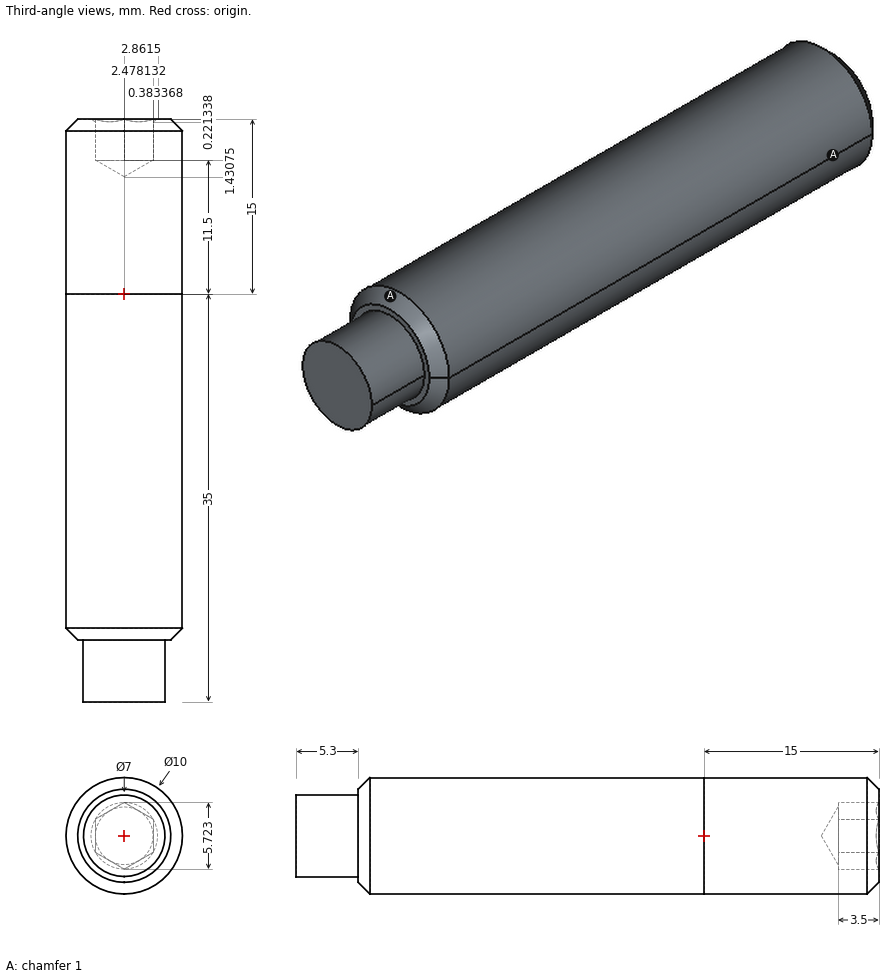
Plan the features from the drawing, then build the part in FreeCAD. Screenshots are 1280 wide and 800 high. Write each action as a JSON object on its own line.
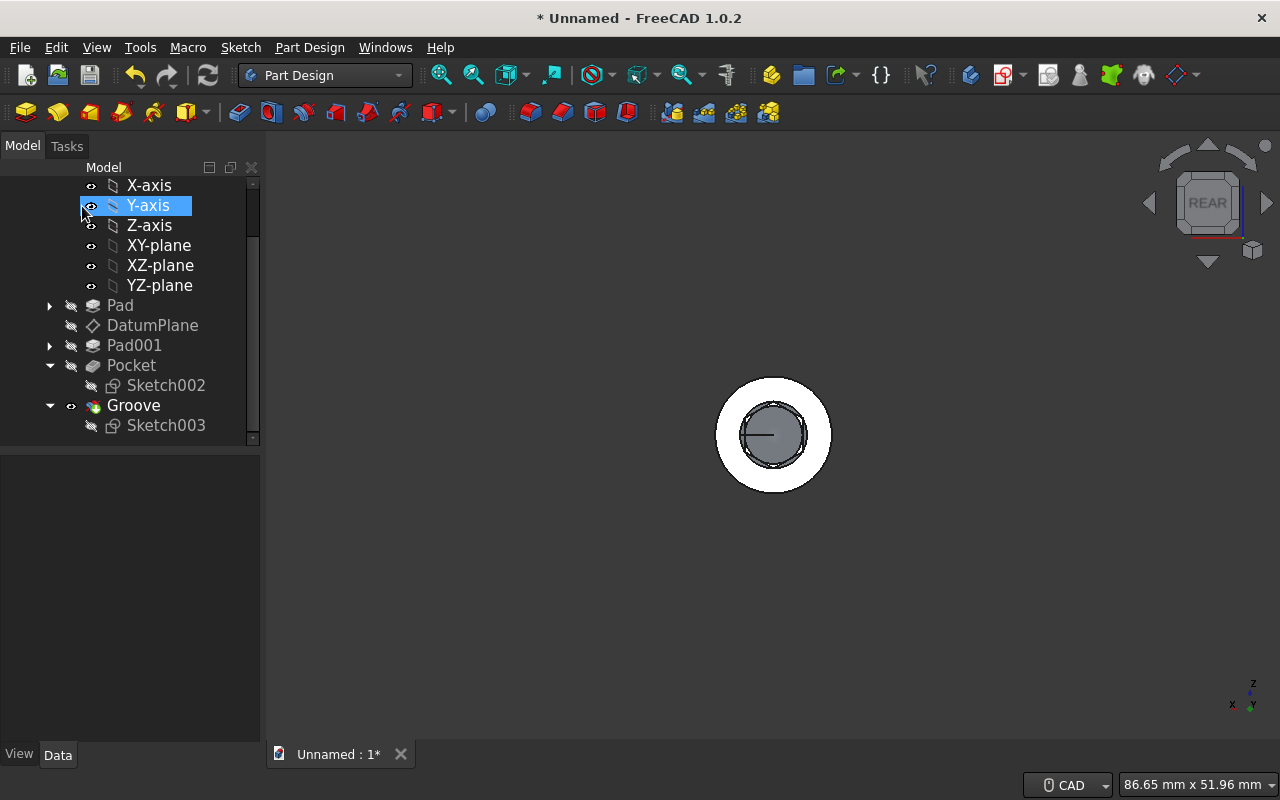
{"action": "left_click", "coordinate": [442, 76]}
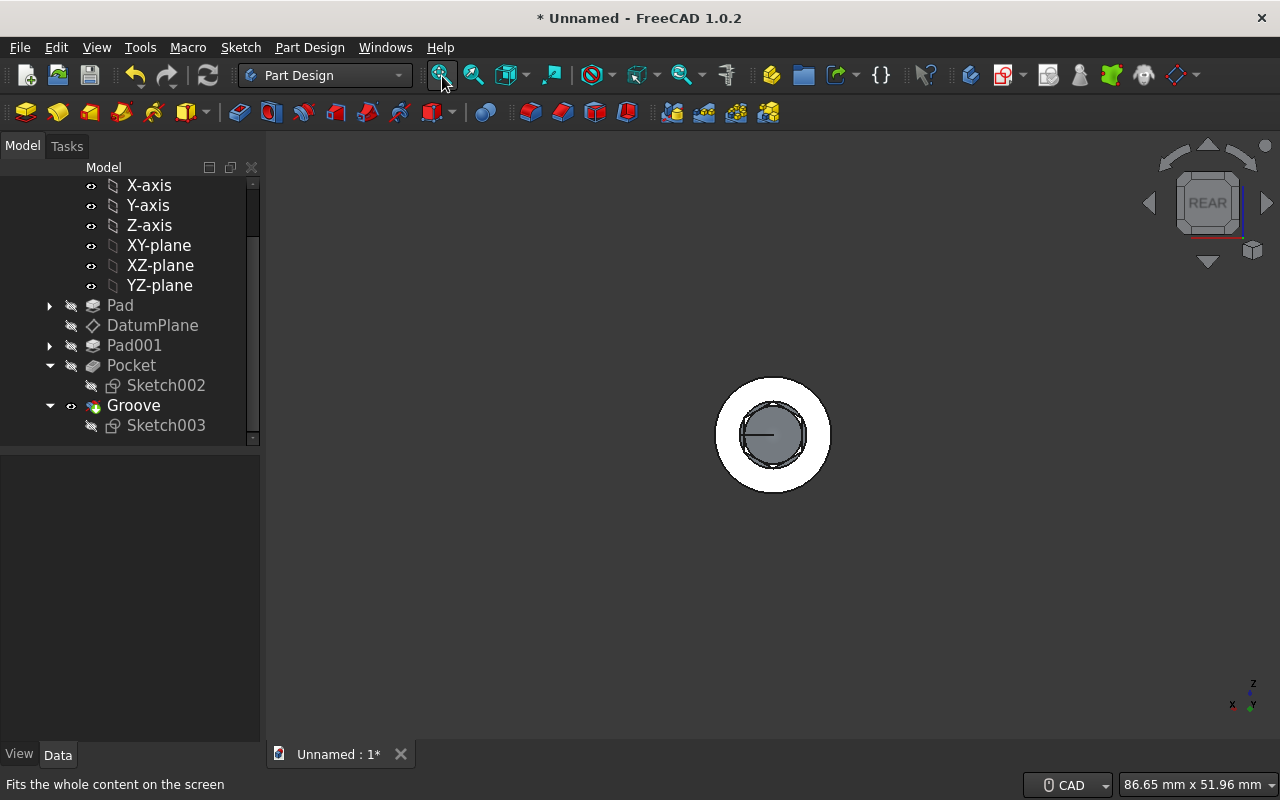
{"action": "key", "text": "0"}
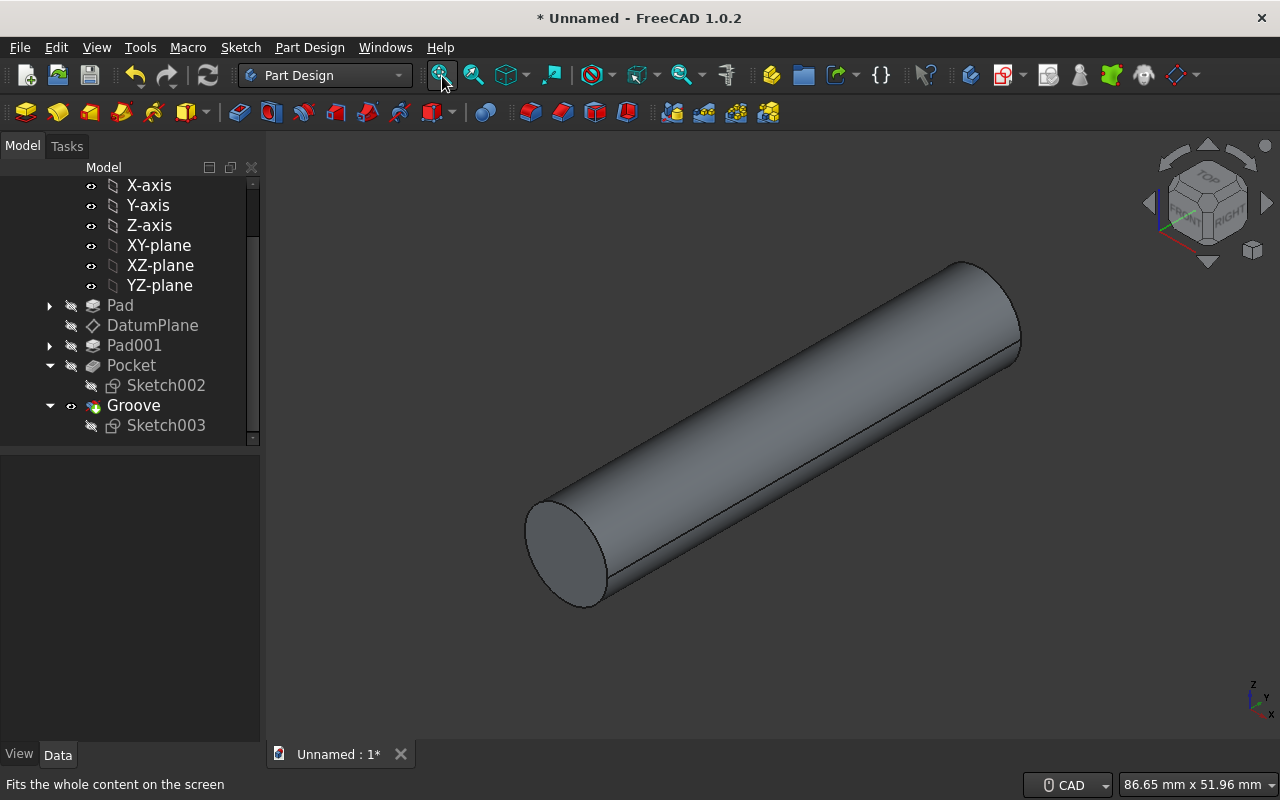
{"action": "left_click", "coordinate": [566, 553]}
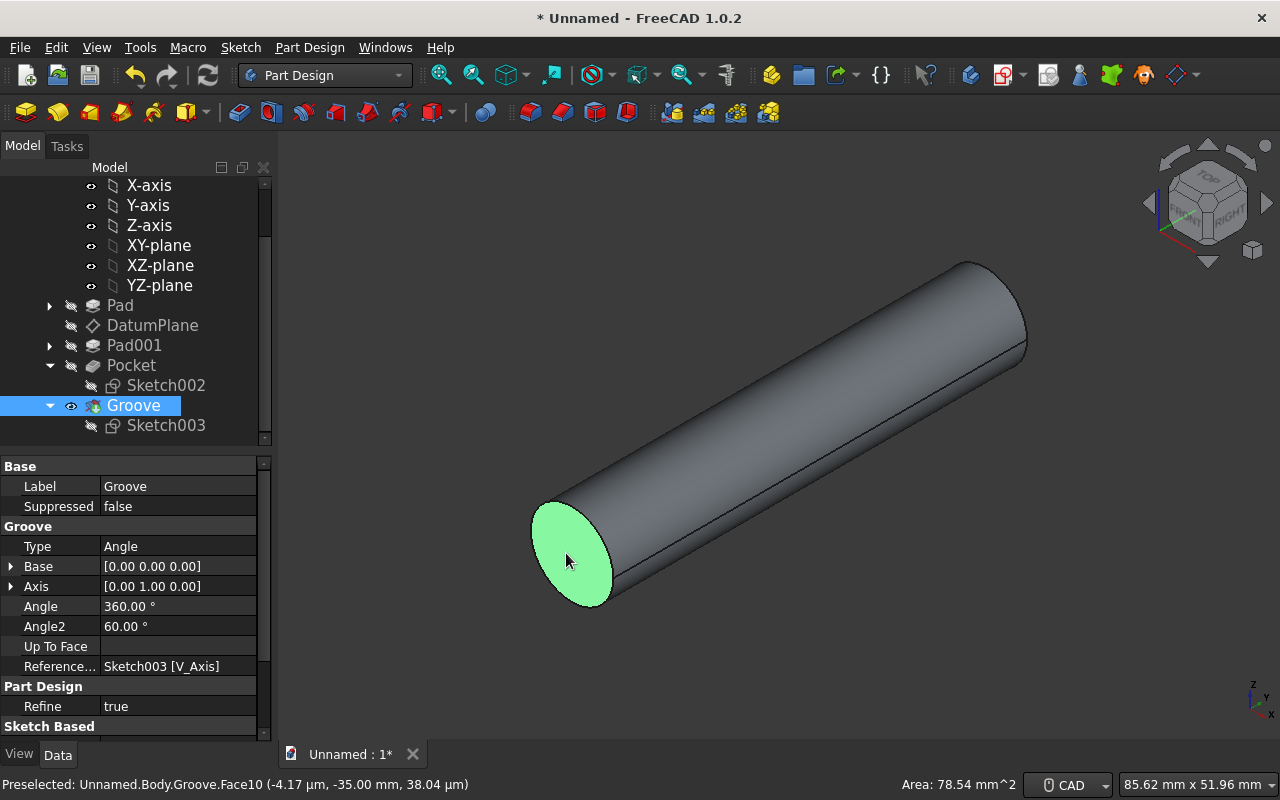
{"action": "left_click", "coordinate": [1004, 76]}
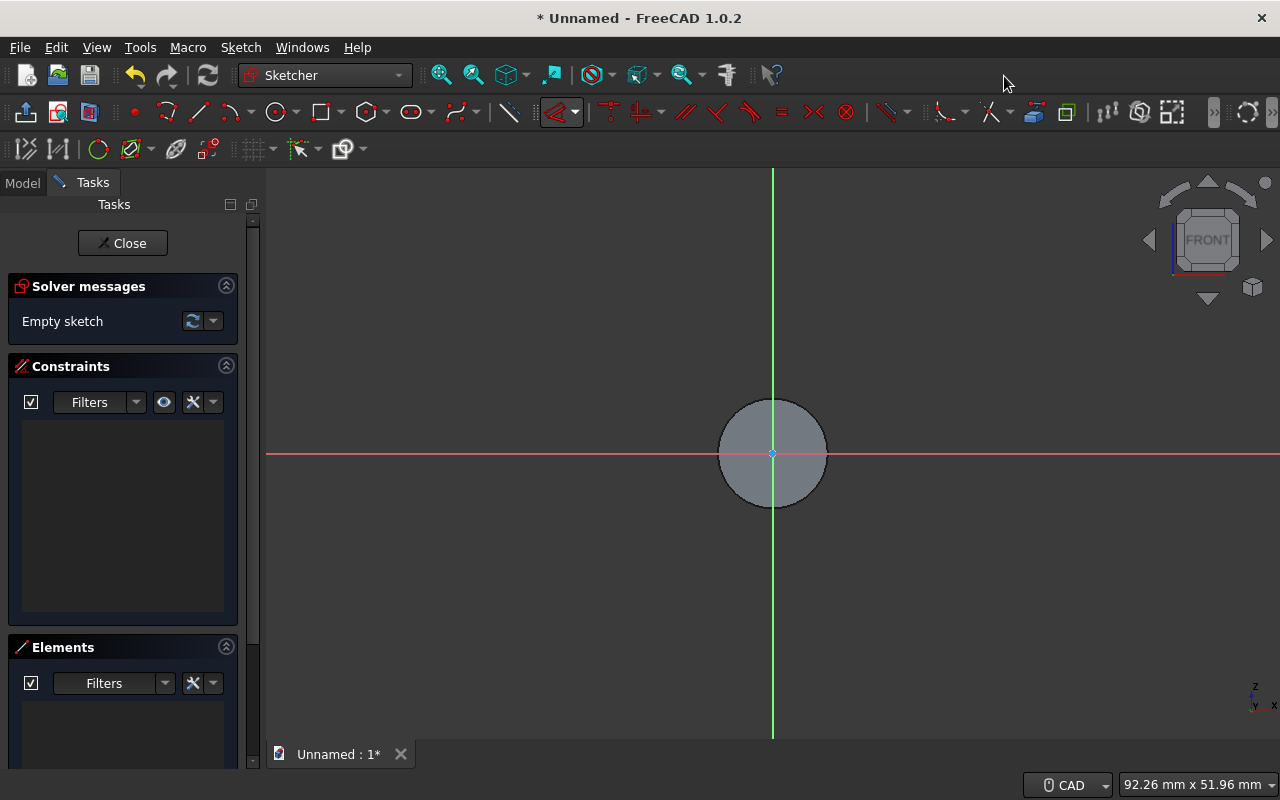
{"action": "scroll", "coordinate": [802, 454], "scroll_direction": "up", "scroll_amount": 6}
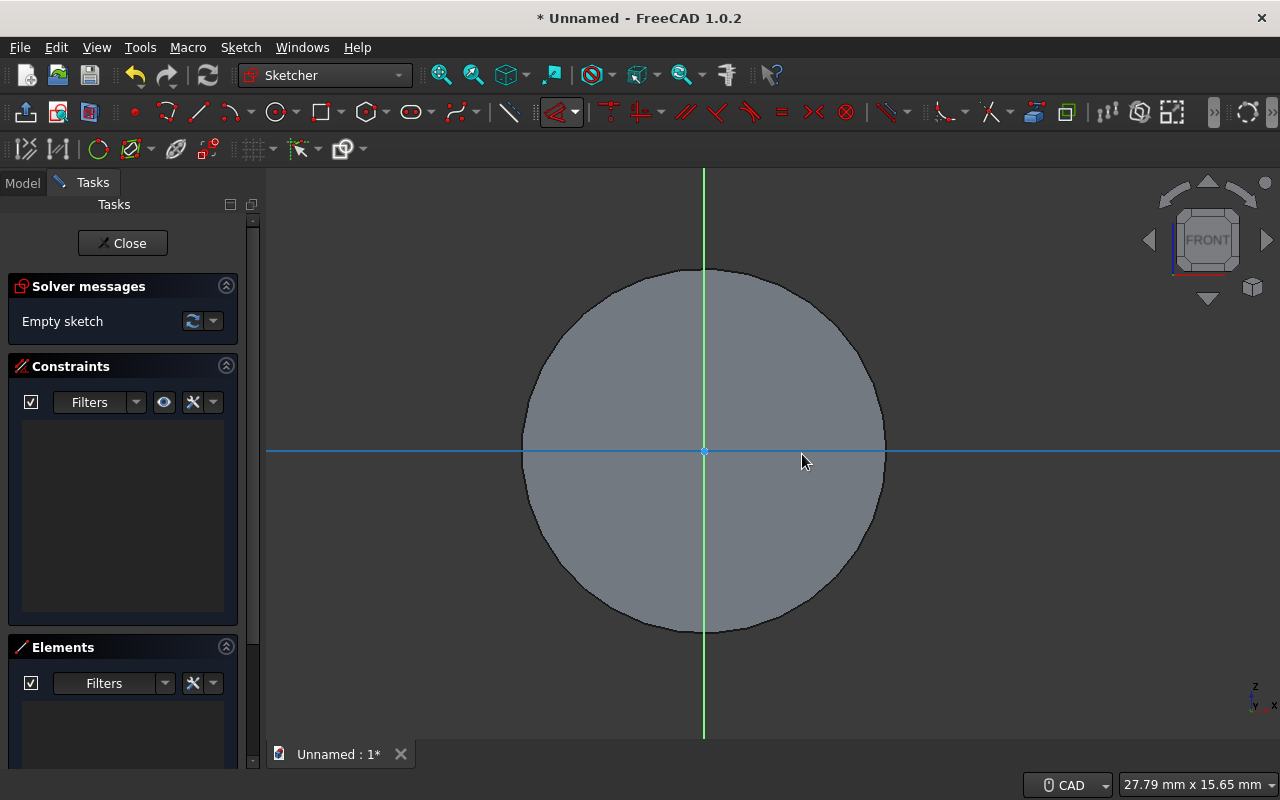
{"action": "left_click", "coordinate": [276, 112]}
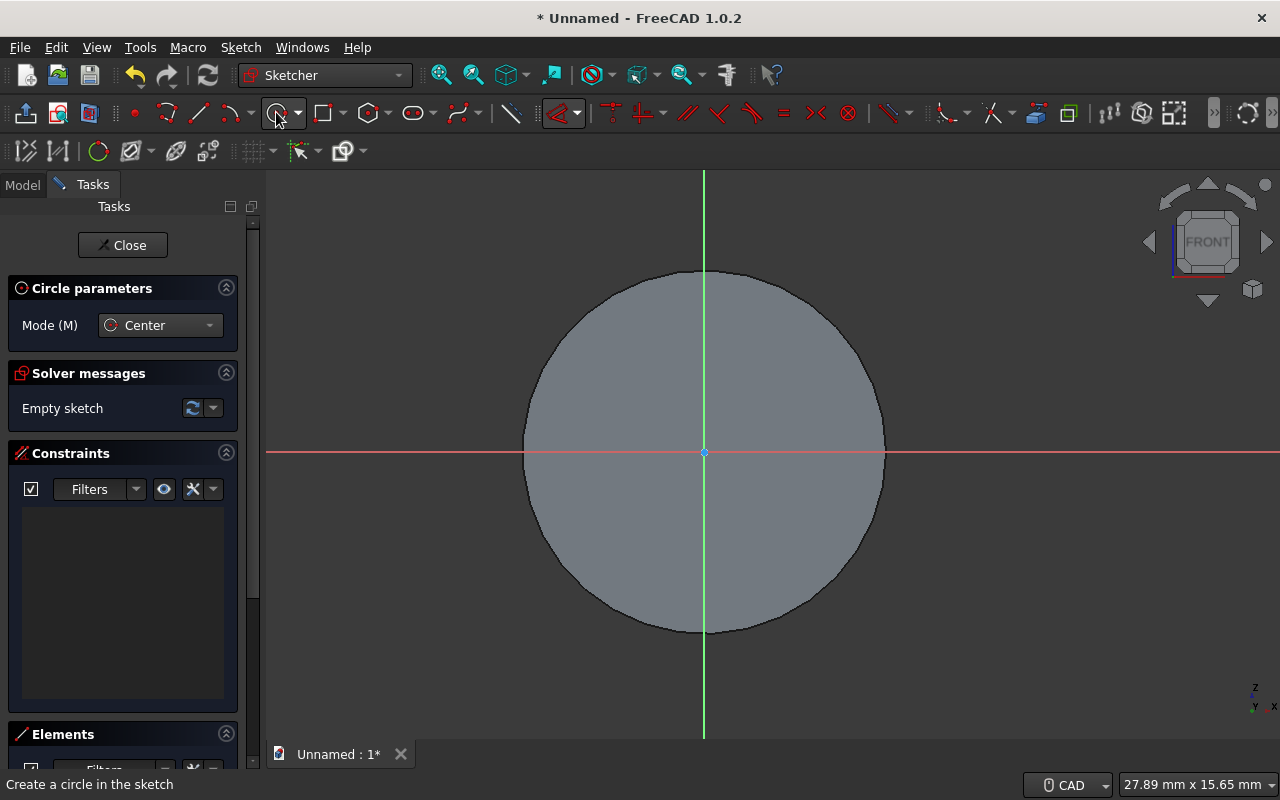
{"action": "left_click", "coordinate": [704, 452]}
{"action": "left_click", "coordinate": [833, 324]}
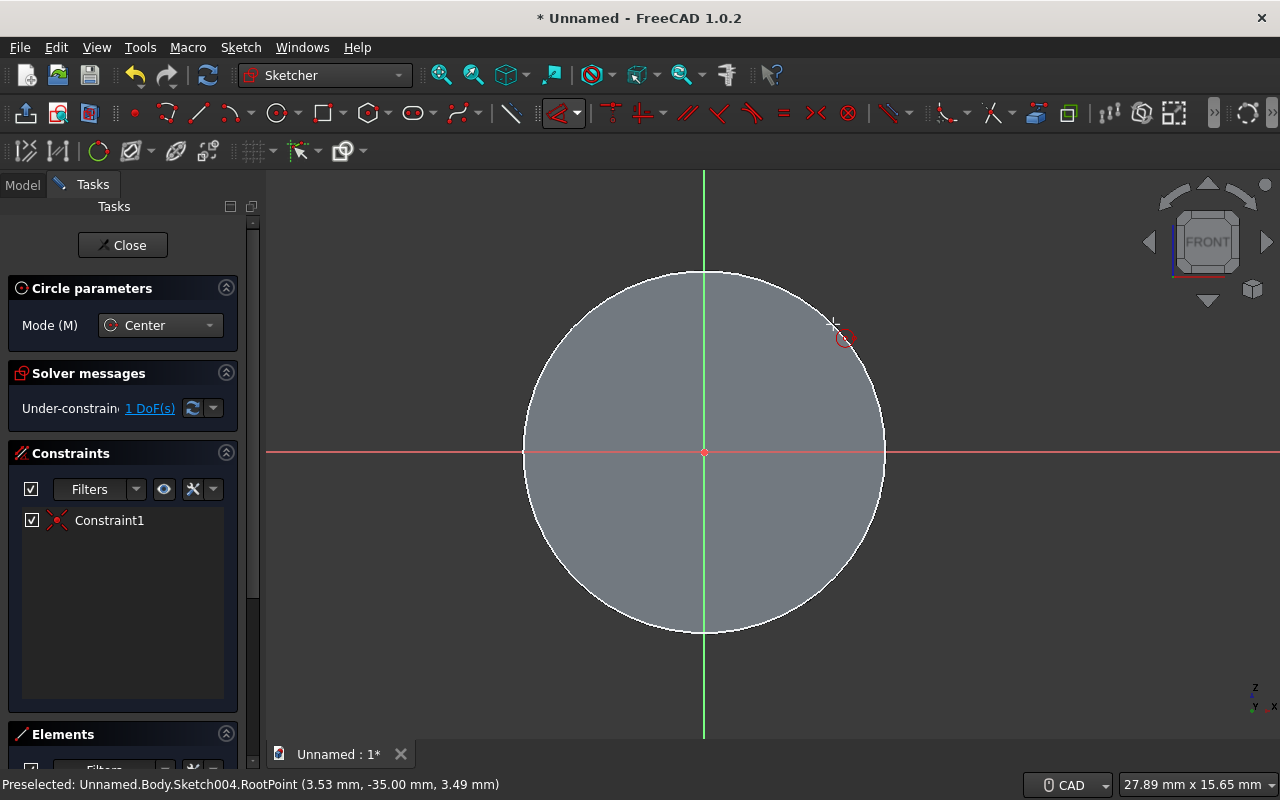
{"action": "left_click", "coordinate": [704, 452]}
{"action": "left_click", "coordinate": [794, 362]}
{"action": "key", "text": "Escape"}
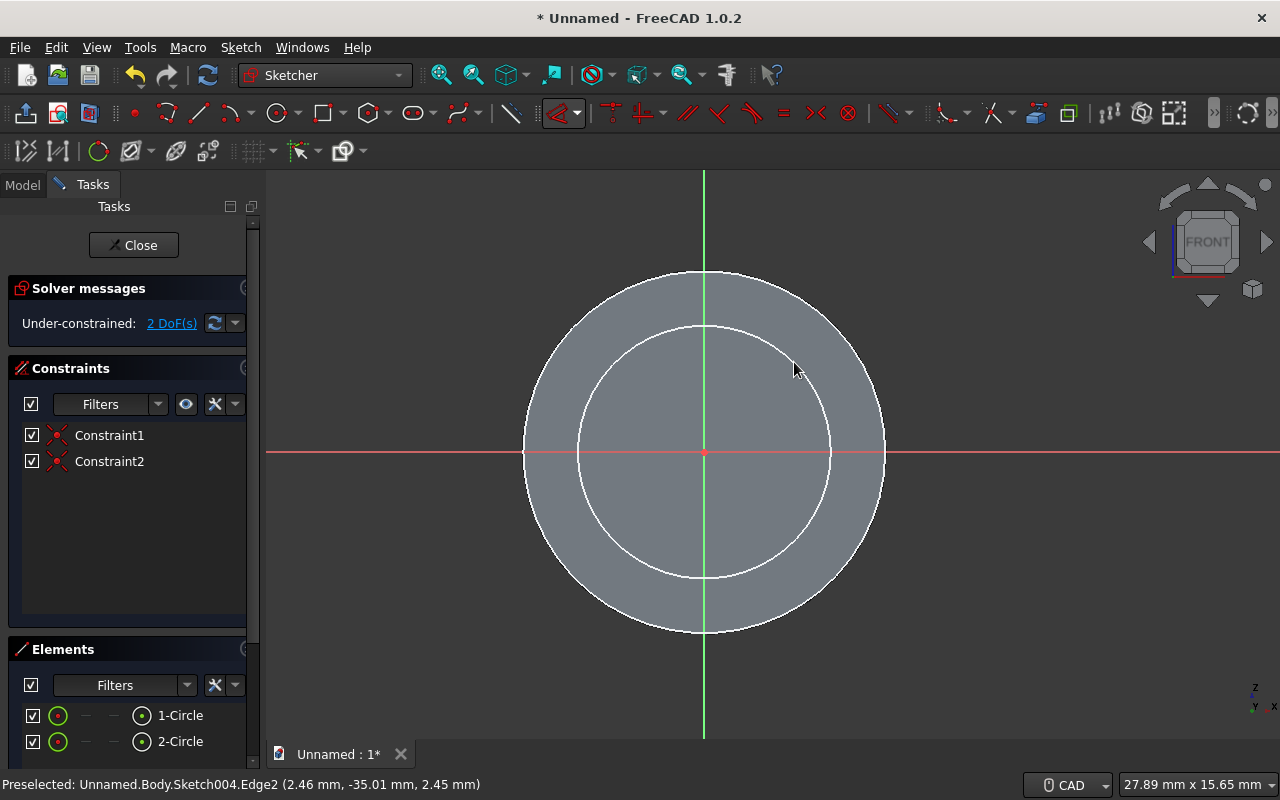
{"action": "left_click", "coordinate": [832, 324]}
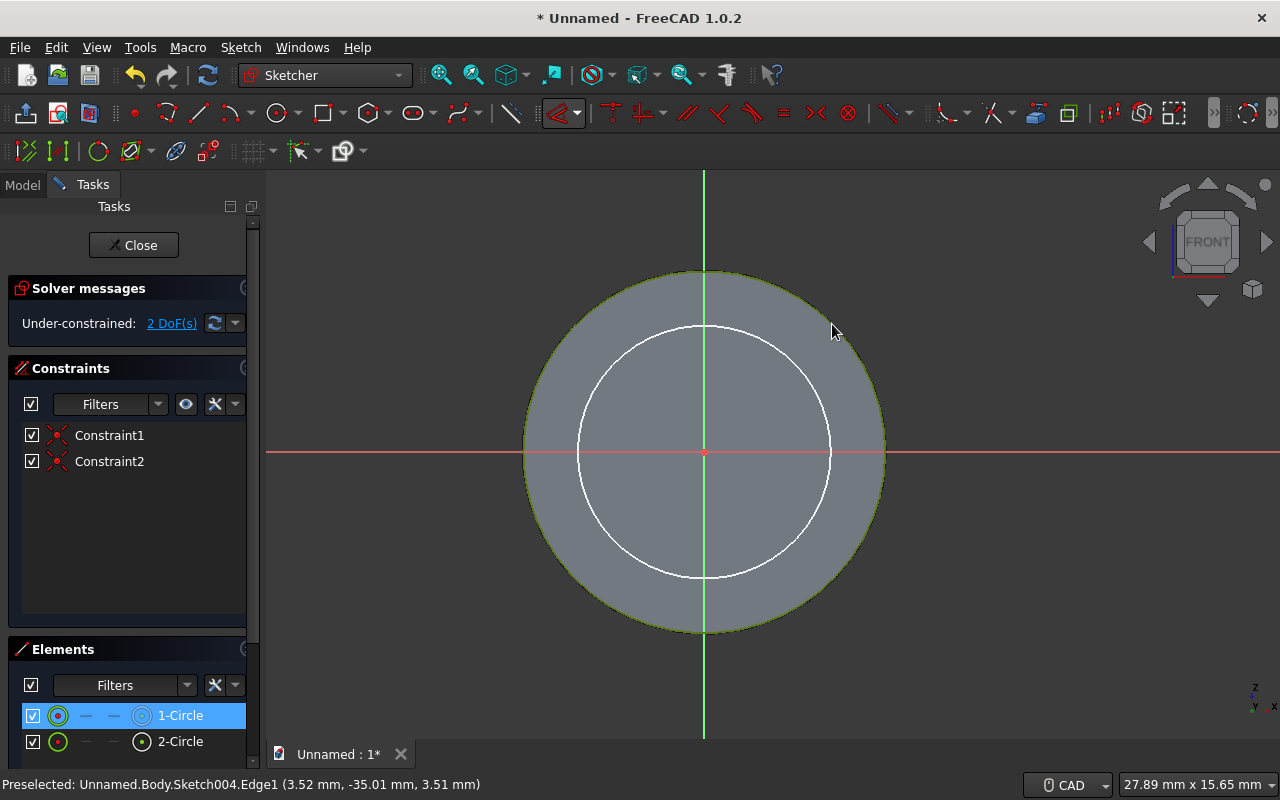
{"action": "key", "text": "k o"}